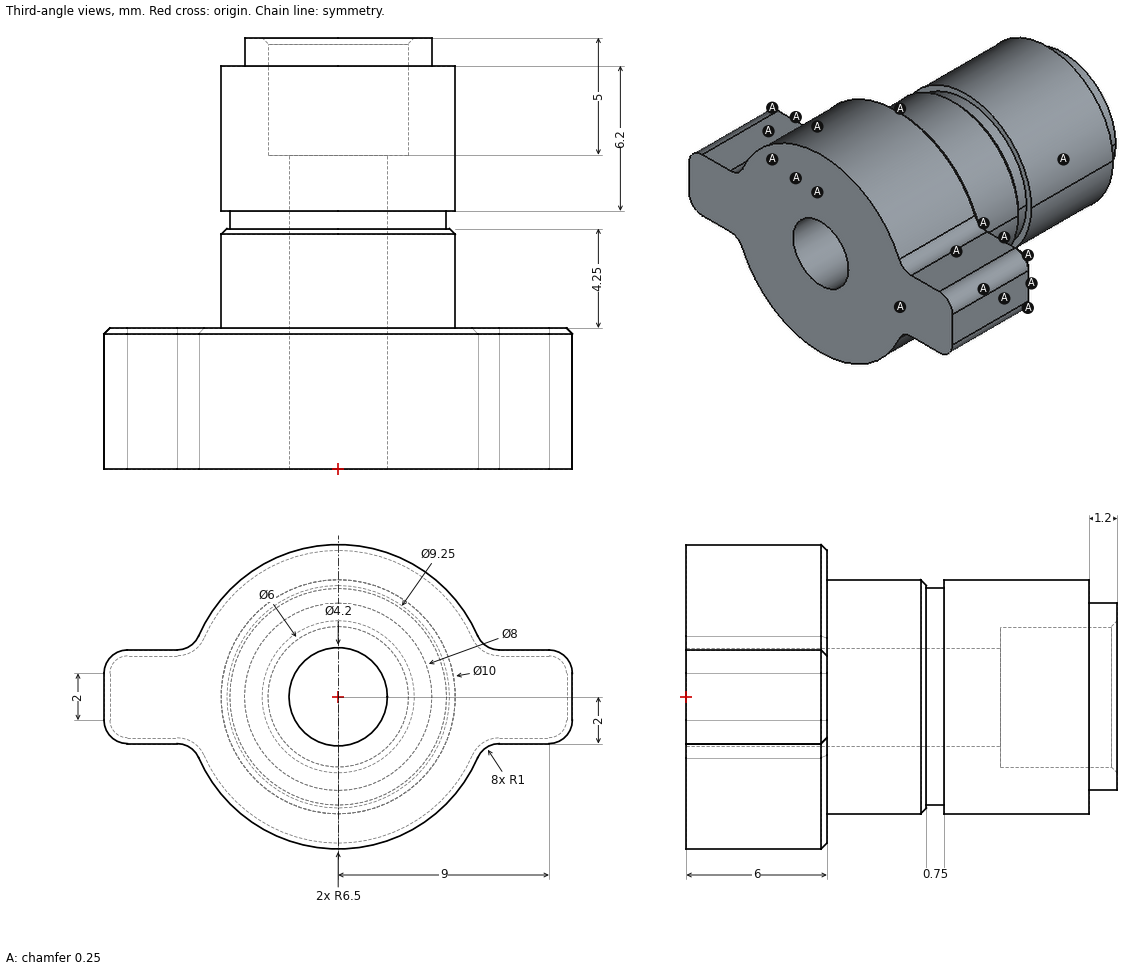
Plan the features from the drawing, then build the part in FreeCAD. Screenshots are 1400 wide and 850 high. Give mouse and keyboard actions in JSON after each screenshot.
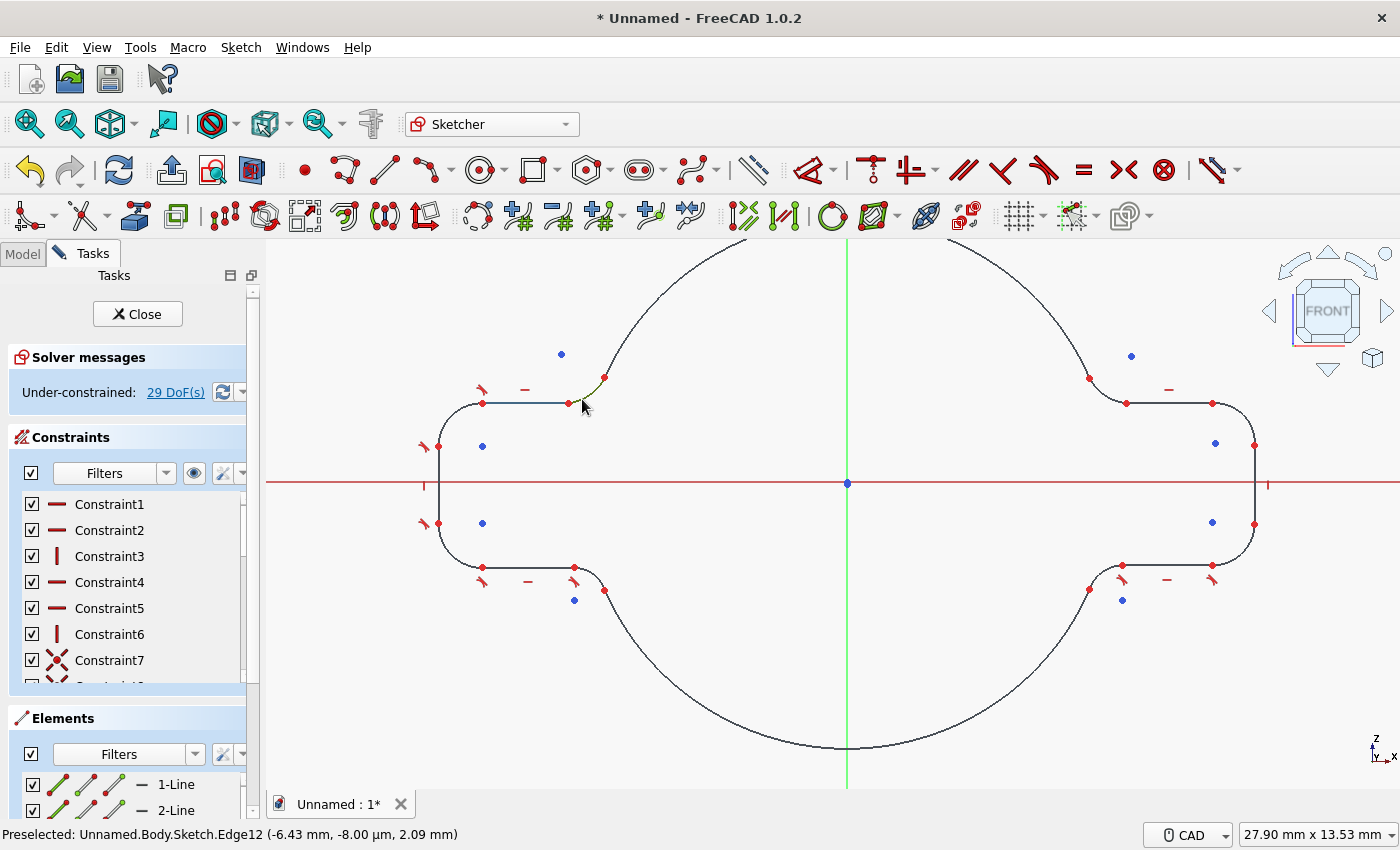
{"action": "left_click", "coordinate": [1044, 170]}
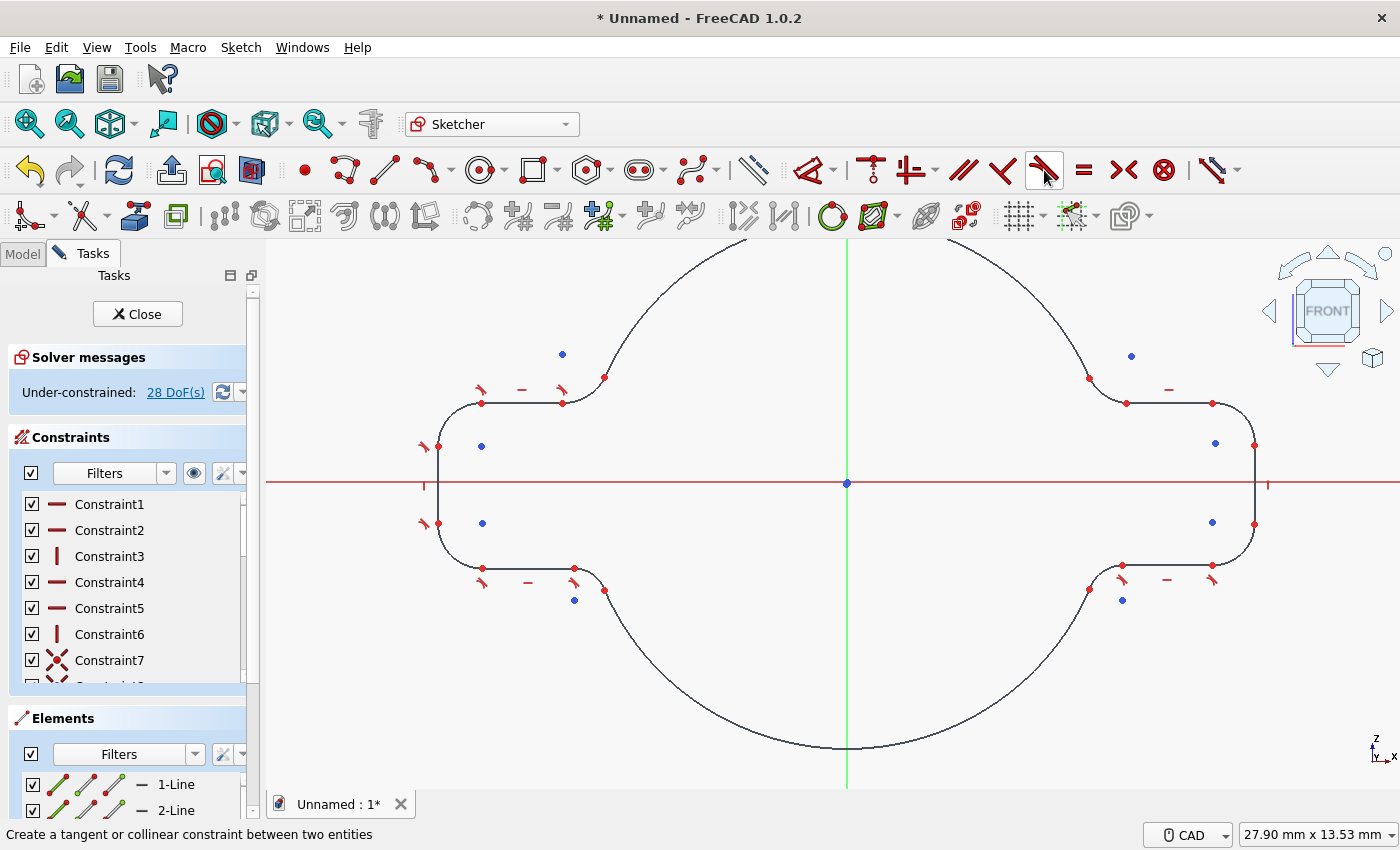
{"action": "left_click", "coordinate": [1152, 403]}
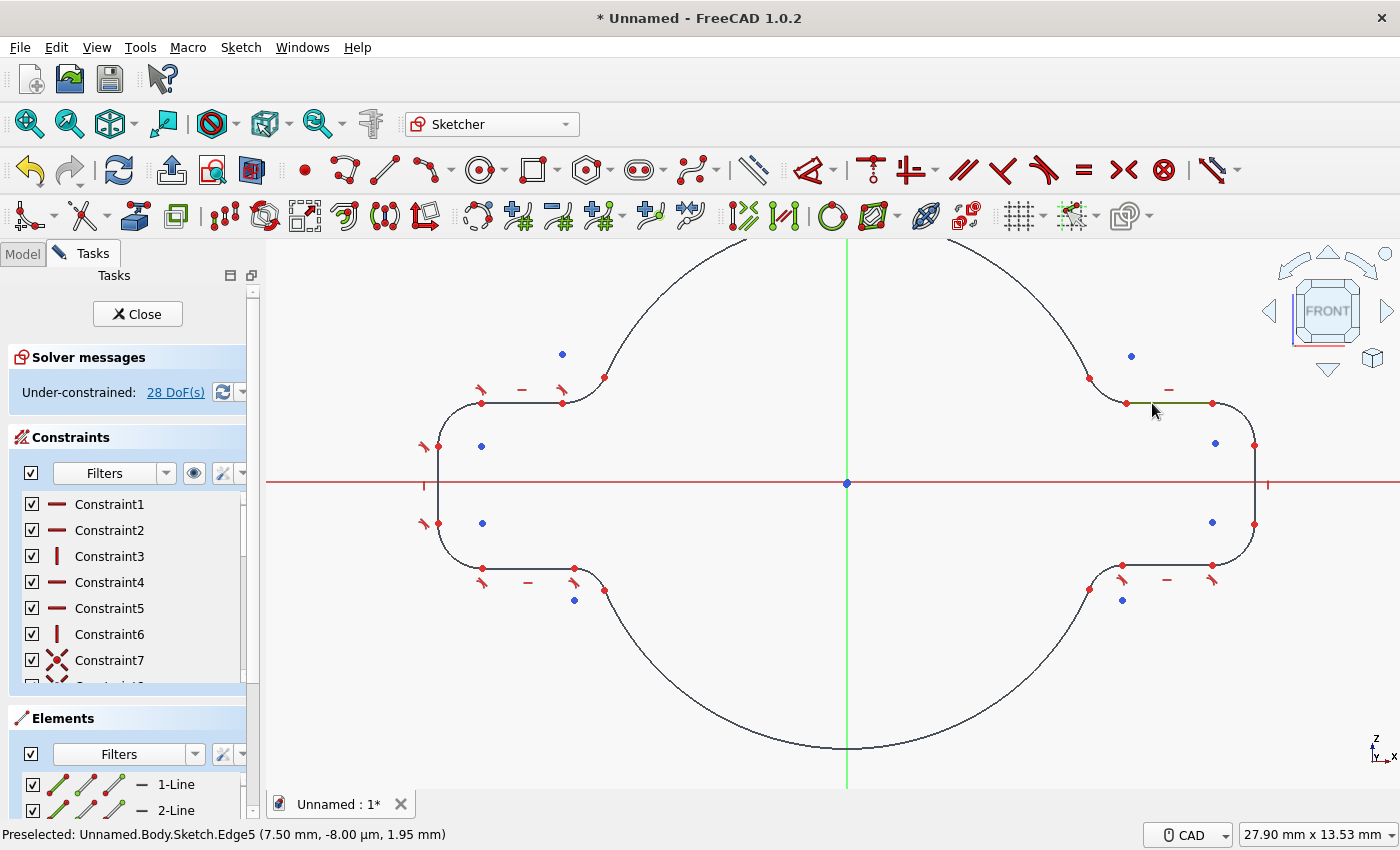
{"action": "left_click", "coordinate": [1098, 390]}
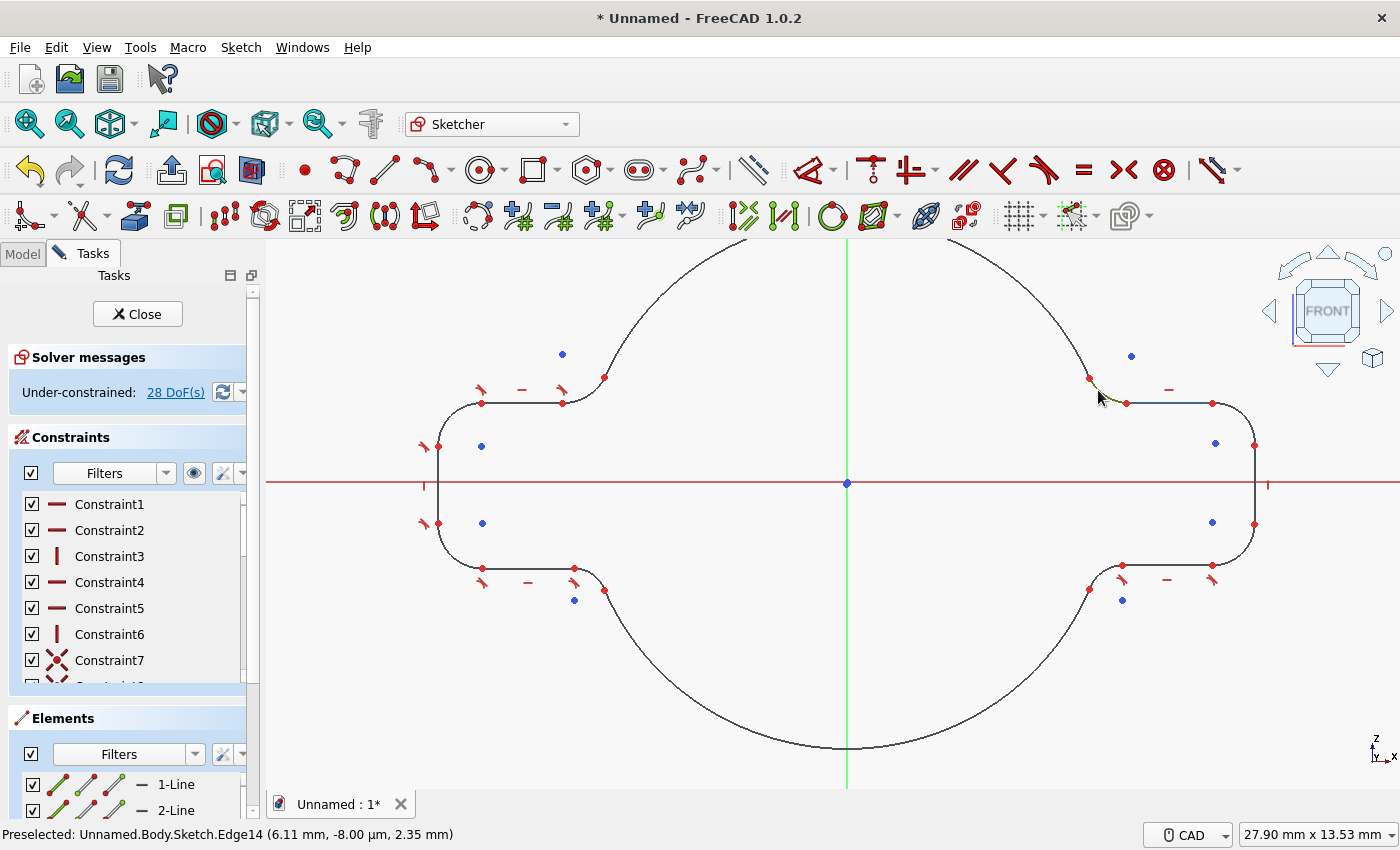
{"action": "left_click", "coordinate": [1044, 170]}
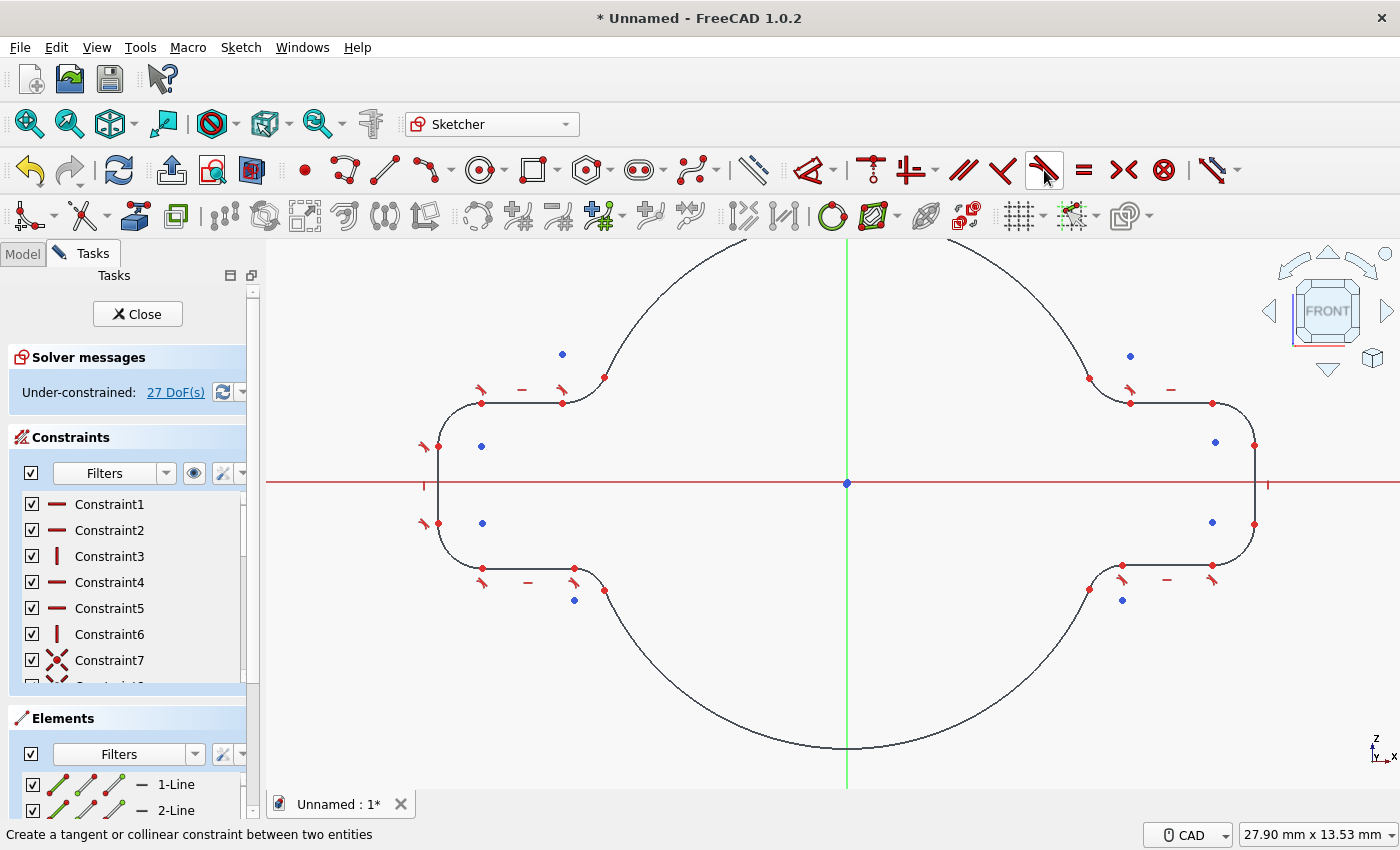
{"action": "left_click", "coordinate": [1156, 403]}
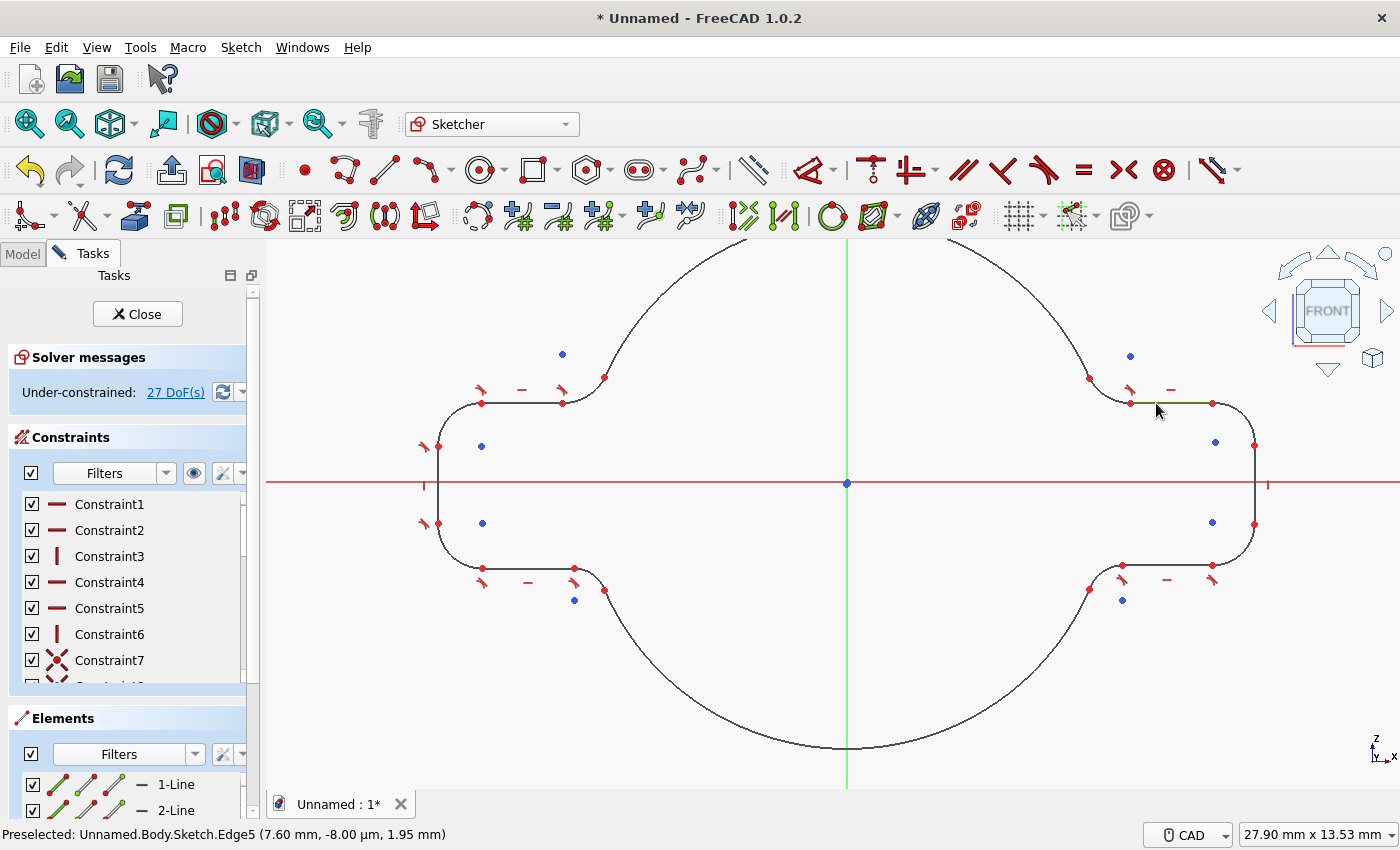
{"action": "left_click", "coordinate": [1232, 407]}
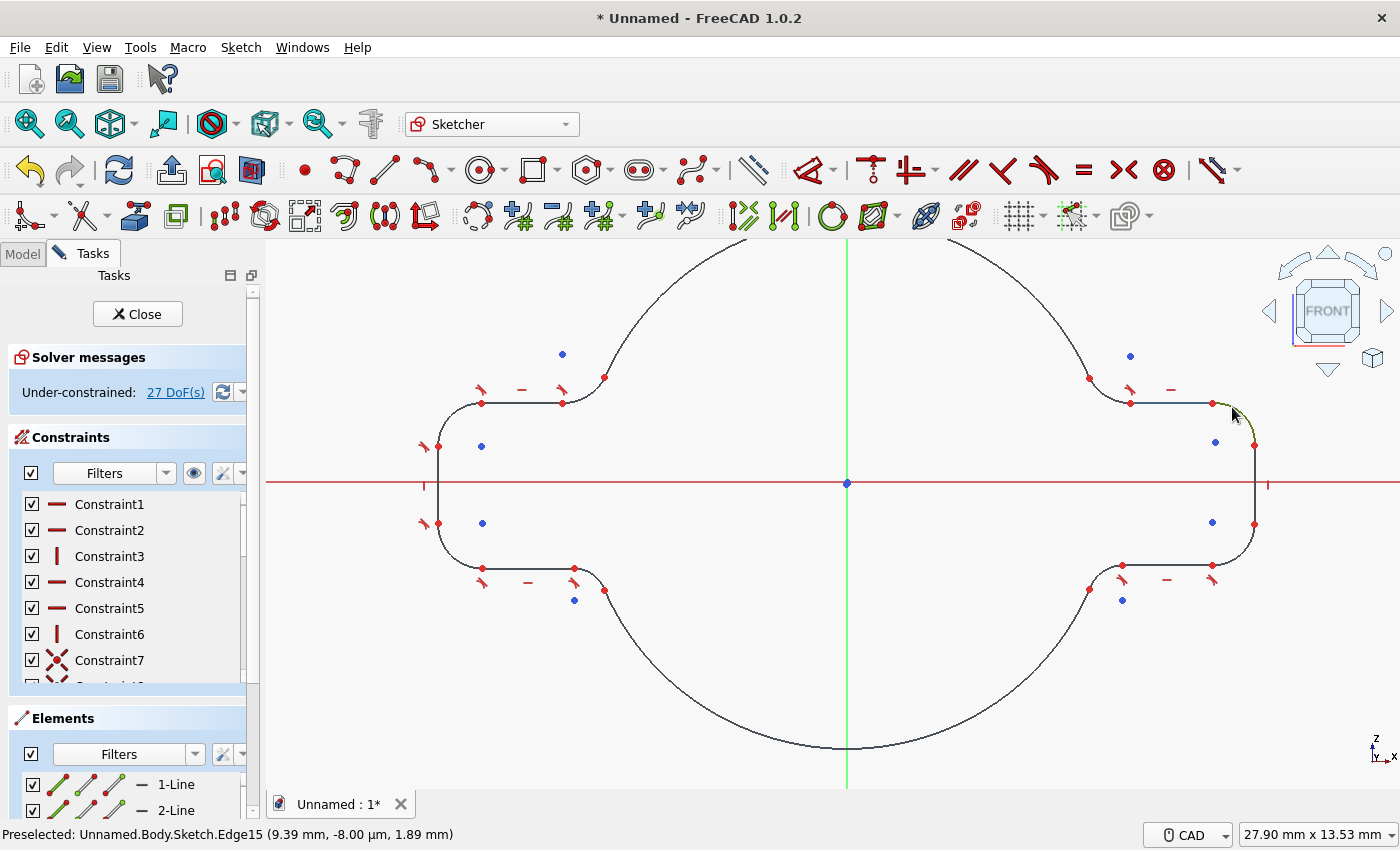
{"action": "left_click", "coordinate": [1044, 170]}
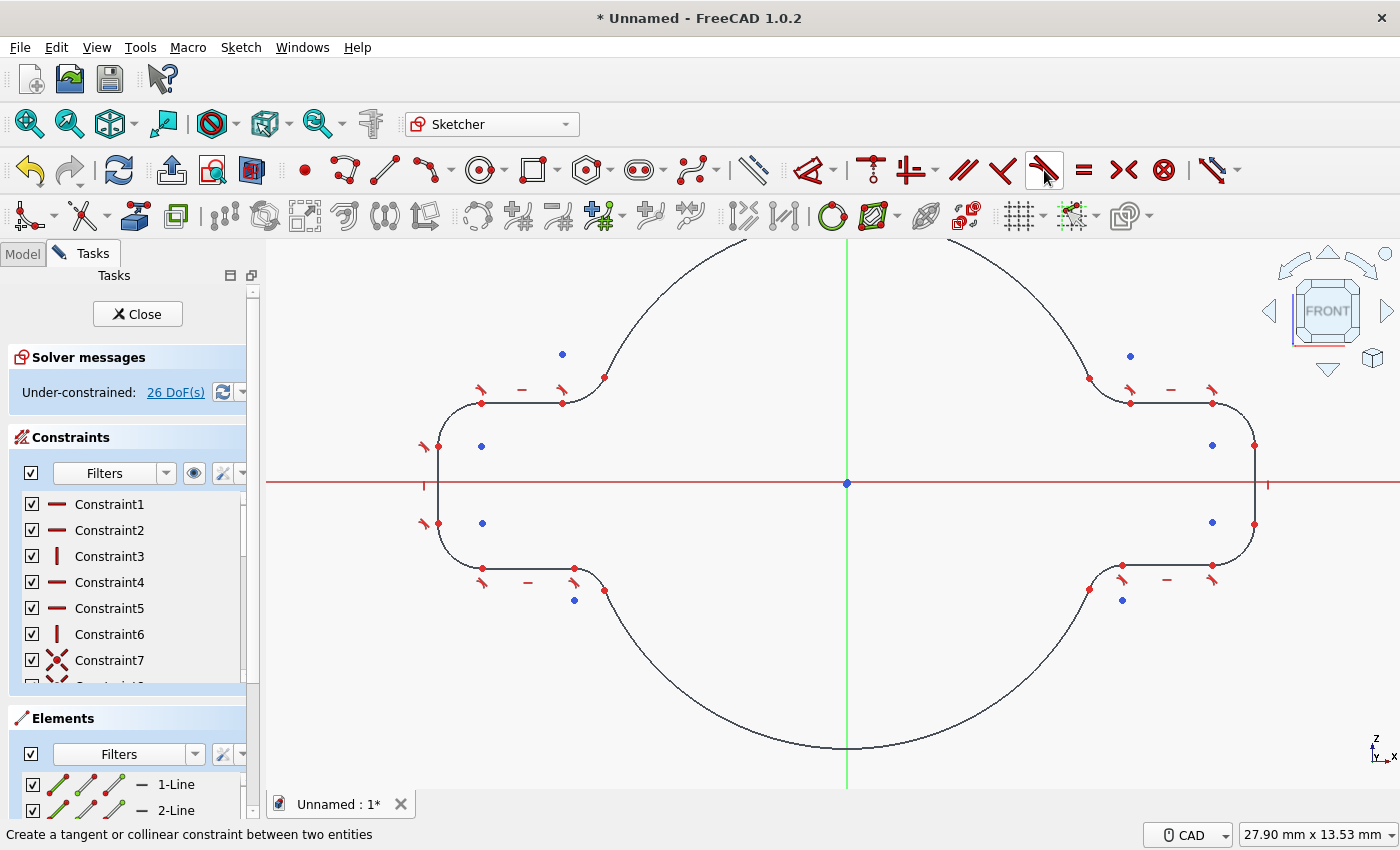
{"action": "scroll", "coordinate": [596, 578], "scroll_direction": "down", "scroll_amount": 2}